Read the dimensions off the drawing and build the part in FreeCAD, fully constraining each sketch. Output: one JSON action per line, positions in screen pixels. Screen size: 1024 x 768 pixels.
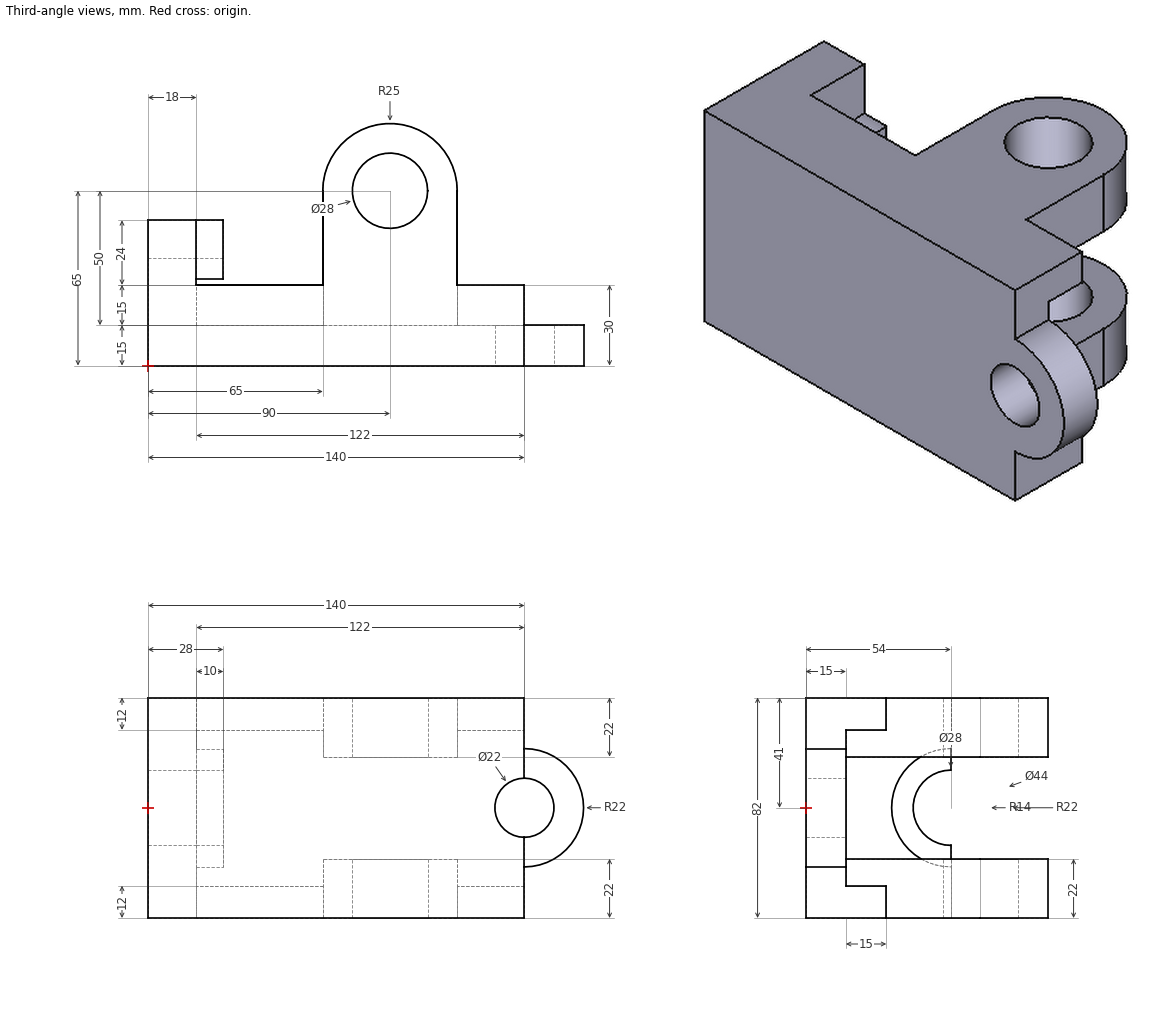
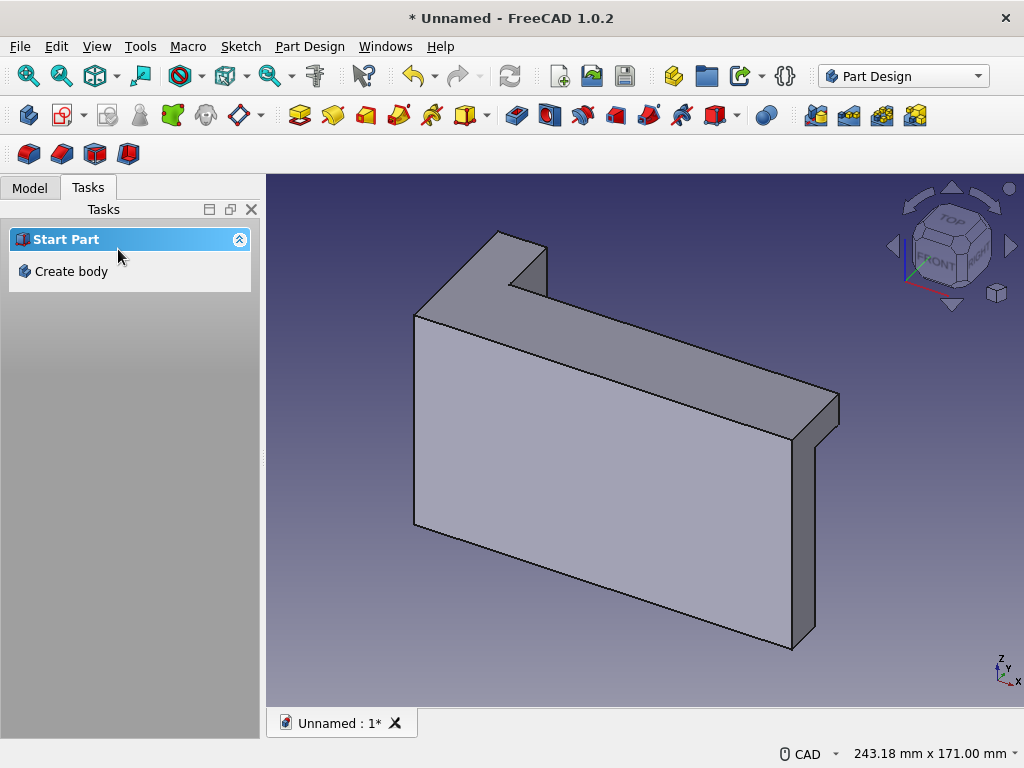
{"action": "key", "text": "5"}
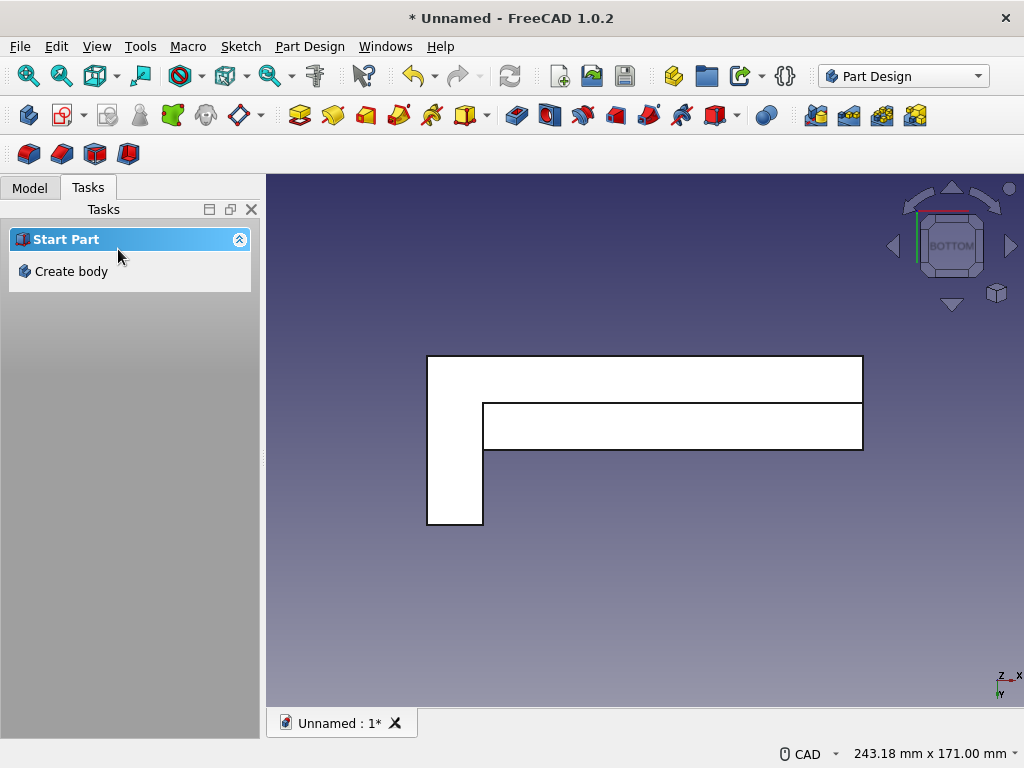
{"action": "left_click", "coordinate": [458, 391]}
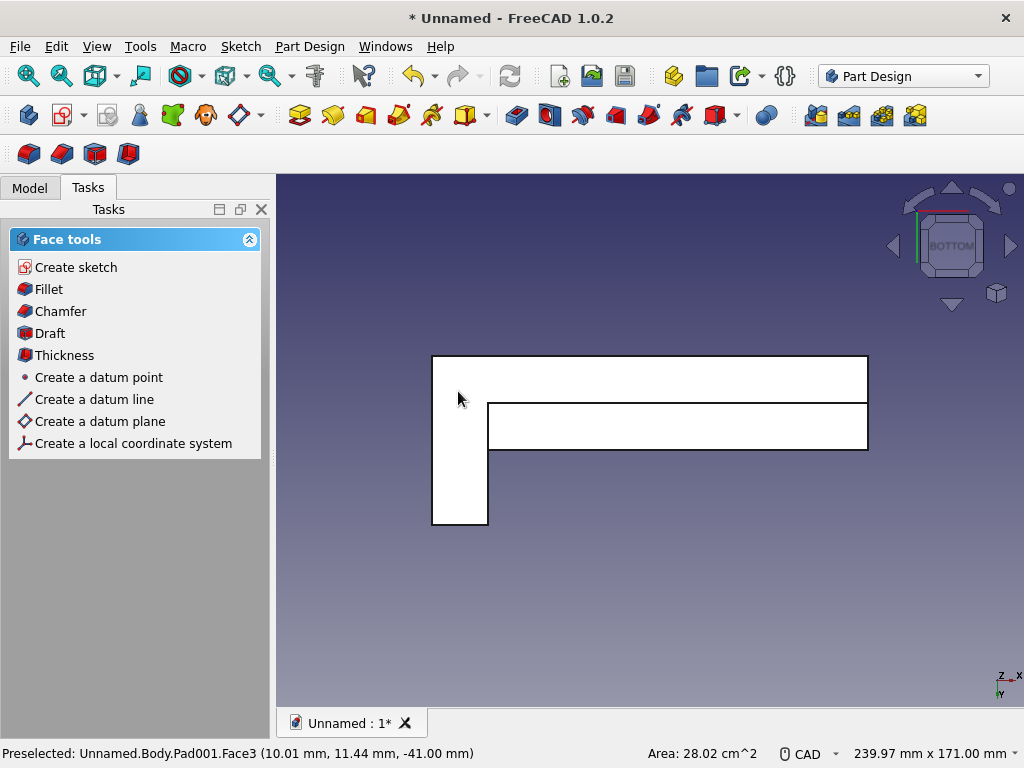
{"action": "left_click", "coordinate": [62, 116]}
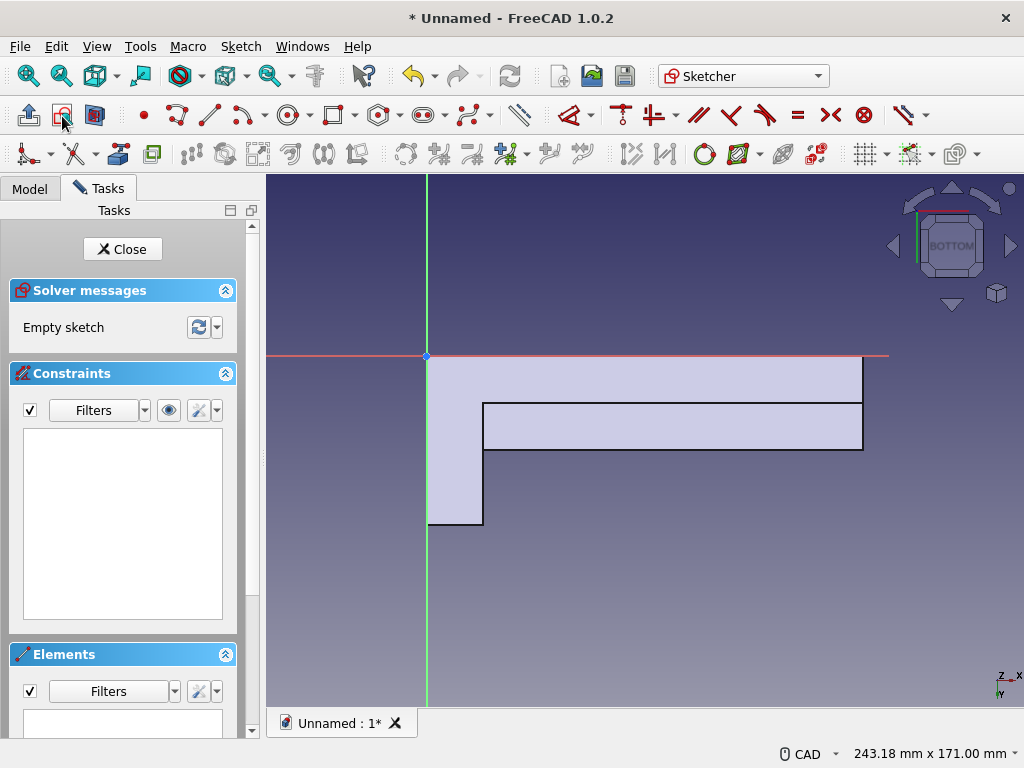
{"action": "scroll", "coordinate": [294, 609], "scroll_direction": "down", "scroll_amount": 1}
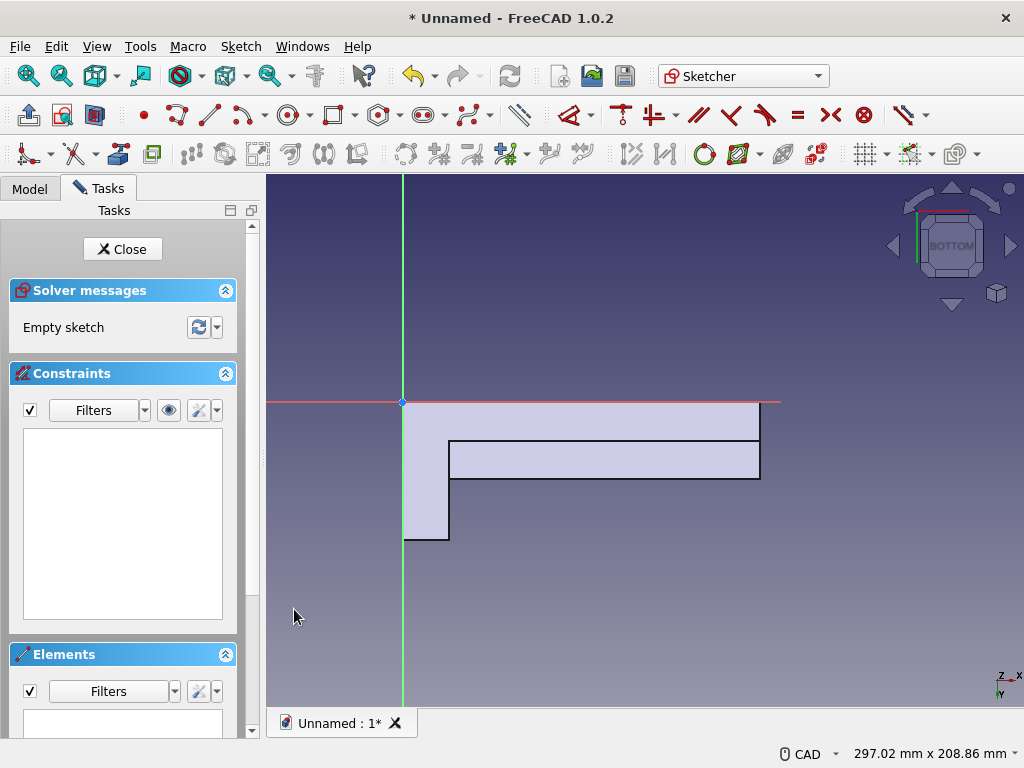
{"action": "key", "text": "g r"}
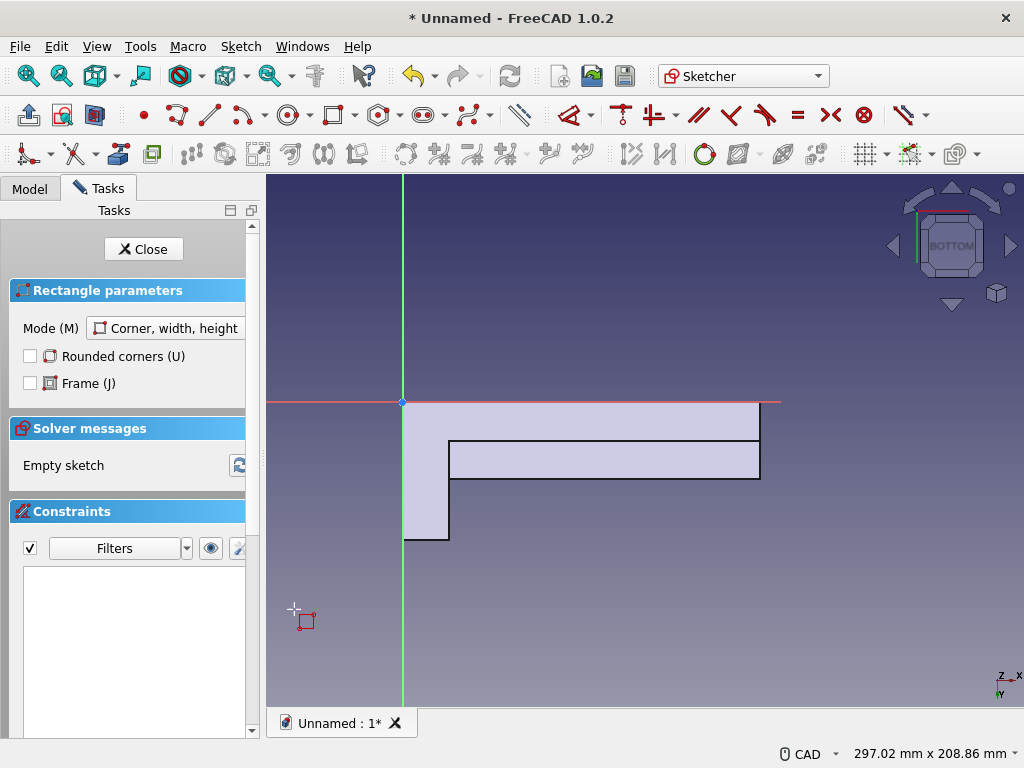
{"action": "left_click", "coordinate": [449, 441]}
{"action": "left_click", "coordinate": [760, 479]}
{"action": "key", "text": "Escape"}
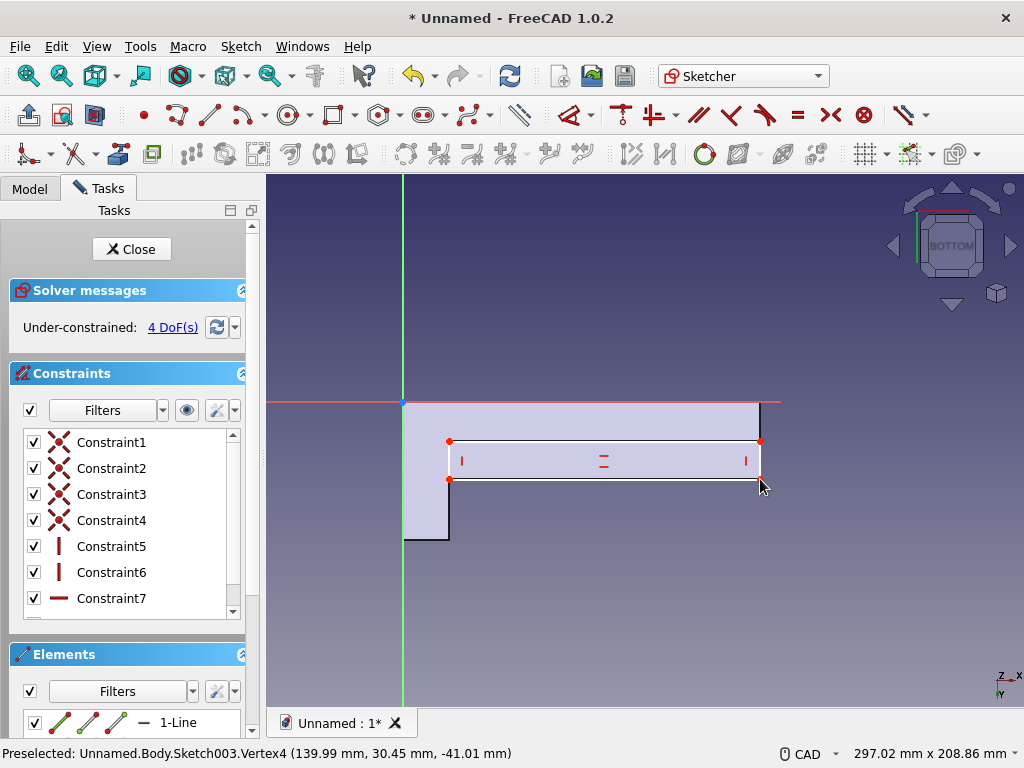
{"action": "key", "text": "d"}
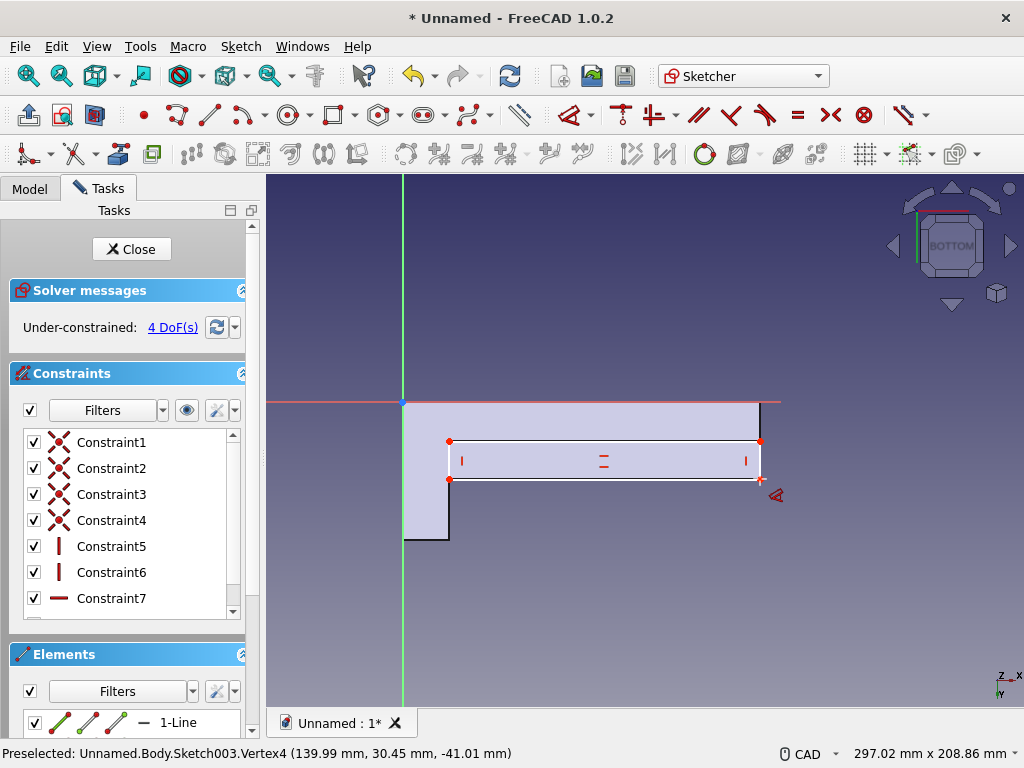
{"action": "left_click", "coordinate": [449, 453]}
{"action": "left_click", "coordinate": [483, 461]}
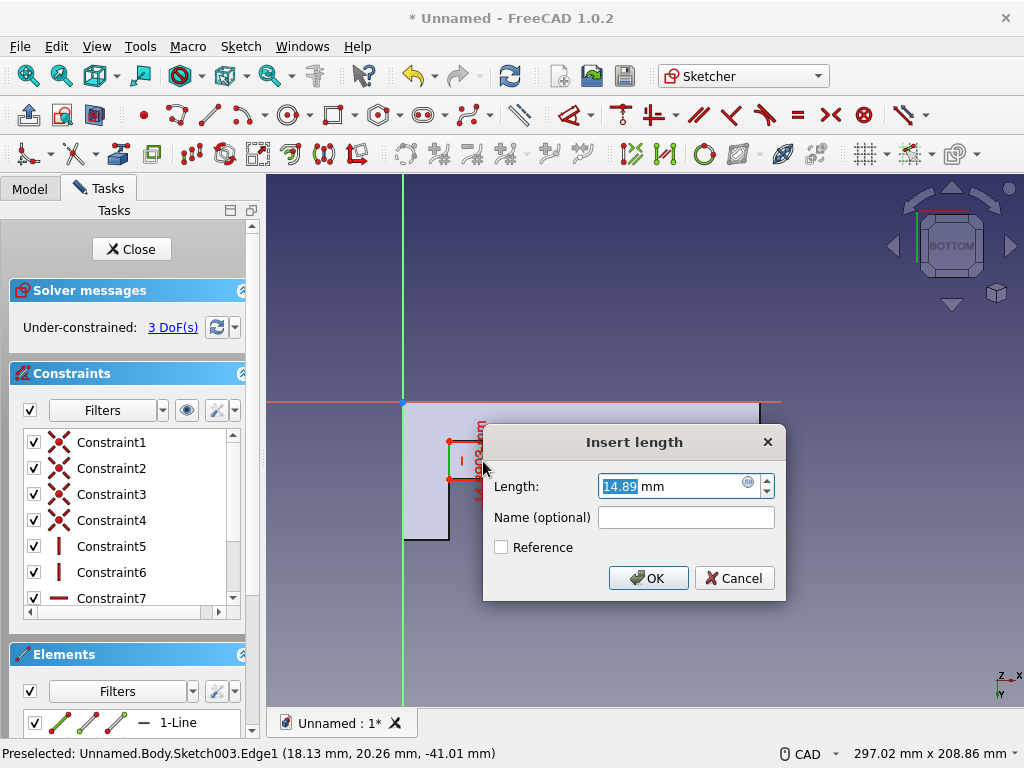
{"action": "type", "text": "15"}
{"action": "key", "text": "Return"}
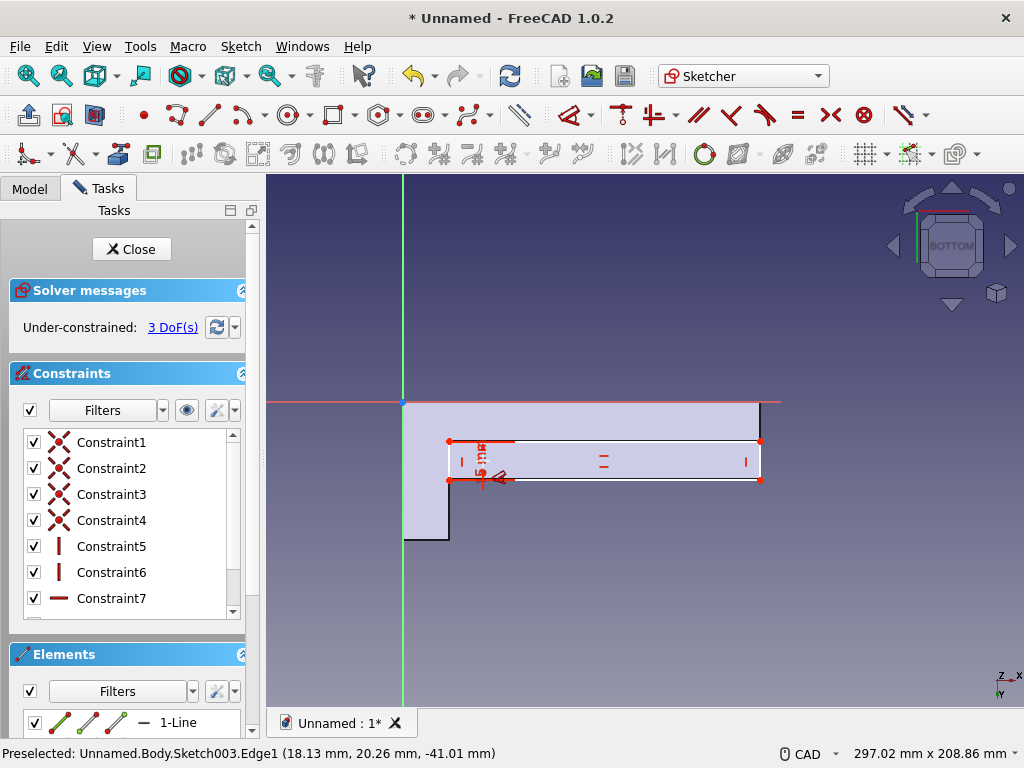
{"action": "left_click", "coordinate": [542, 480]}
{"action": "left_click", "coordinate": [605, 514]}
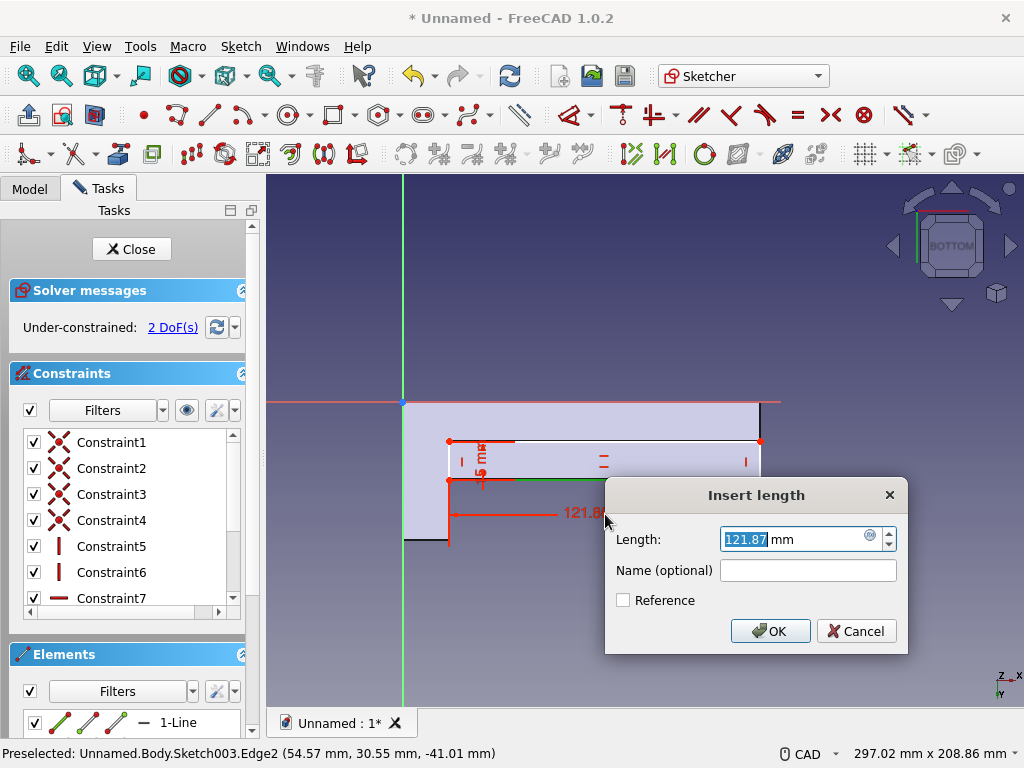
{"action": "type", "text": "122"}
{"action": "key", "text": "Return"}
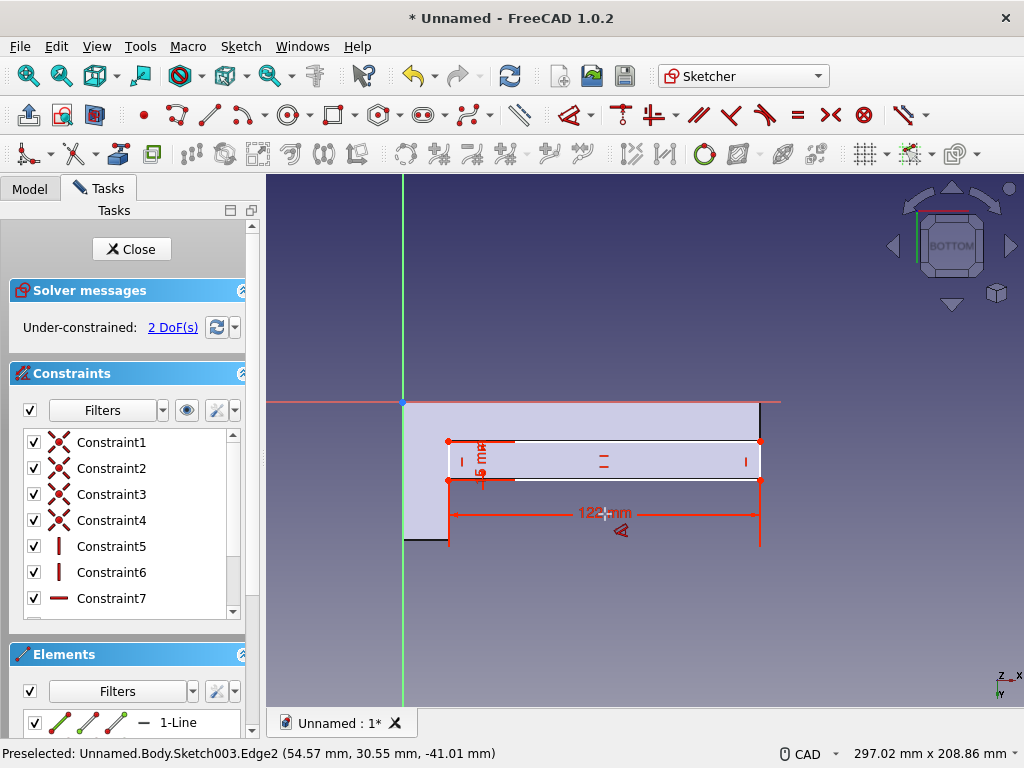
{"action": "left_click", "coordinate": [449, 442]}
{"action": "left_click", "coordinate": [426, 368]}